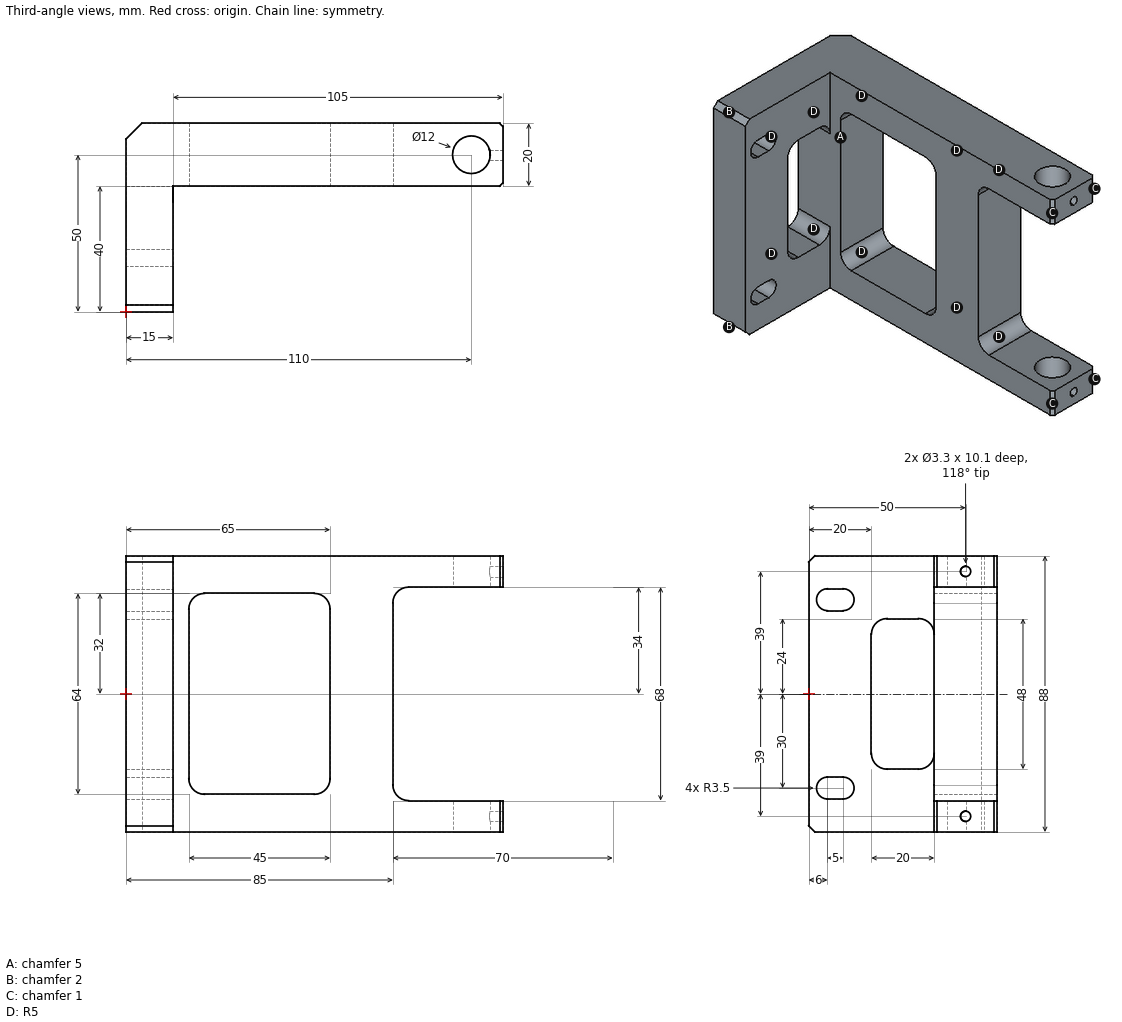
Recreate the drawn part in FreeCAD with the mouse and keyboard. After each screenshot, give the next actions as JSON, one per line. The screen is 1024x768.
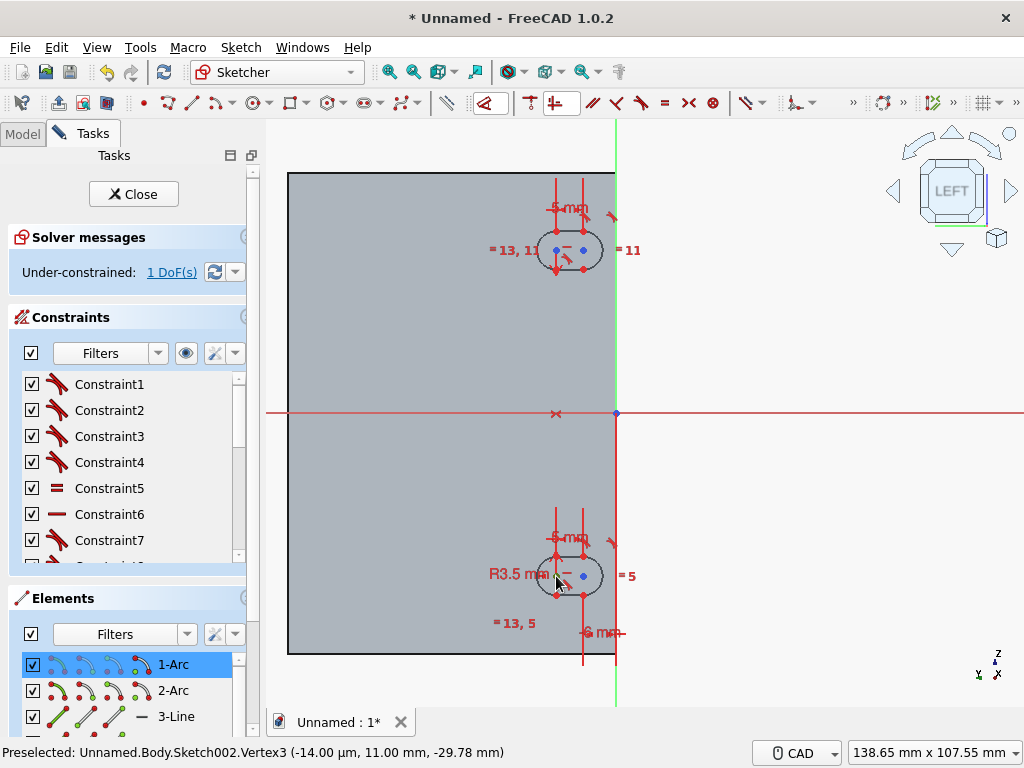
{"action": "key", "text": "i"}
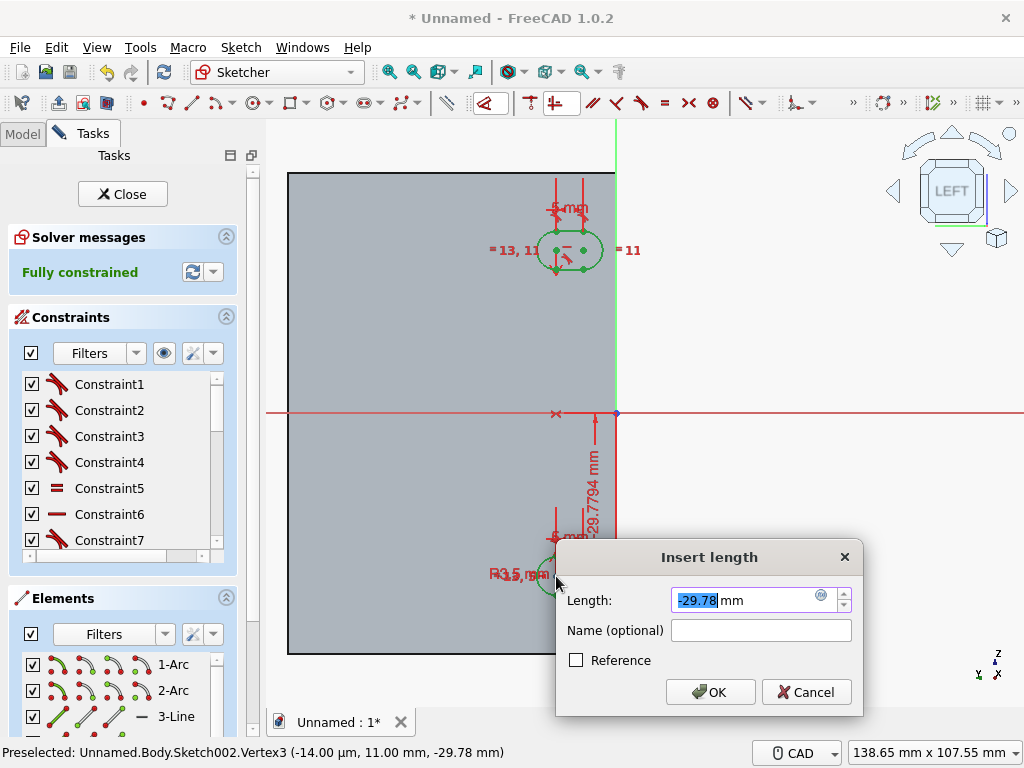
{"action": "type", "text": "-30"}
{"action": "key", "text": "Return"}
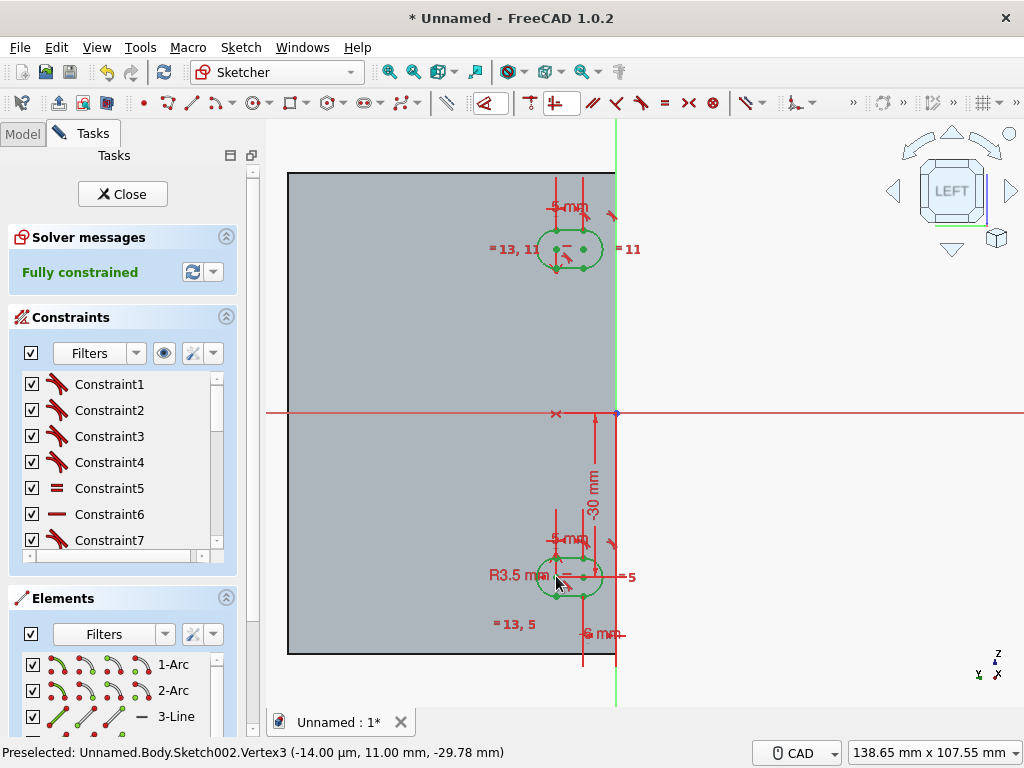
{"action": "left_click", "coordinate": [123, 194]}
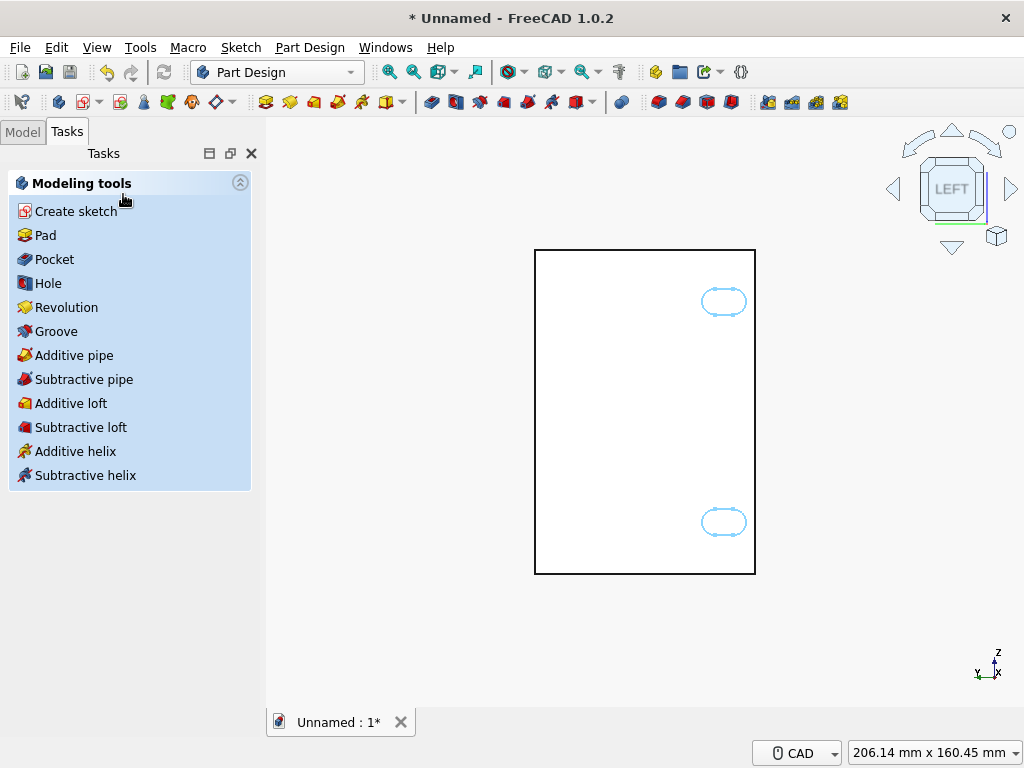
{"action": "left_click", "coordinate": [432, 102]}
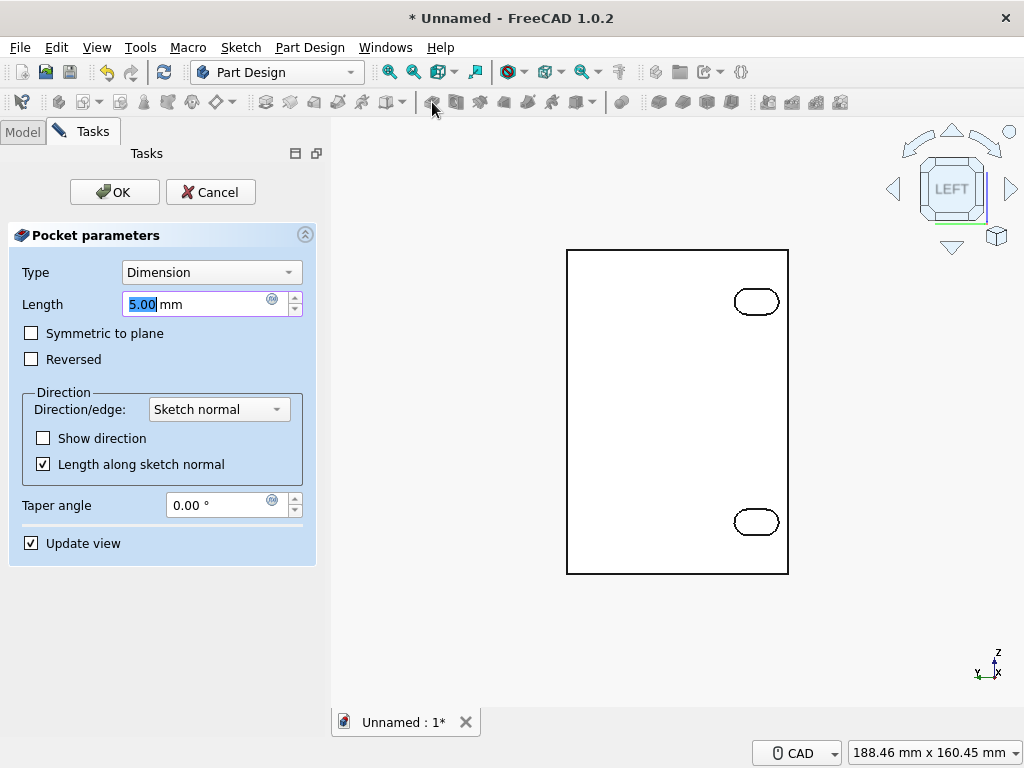
{"action": "left_click", "coordinate": [212, 272]}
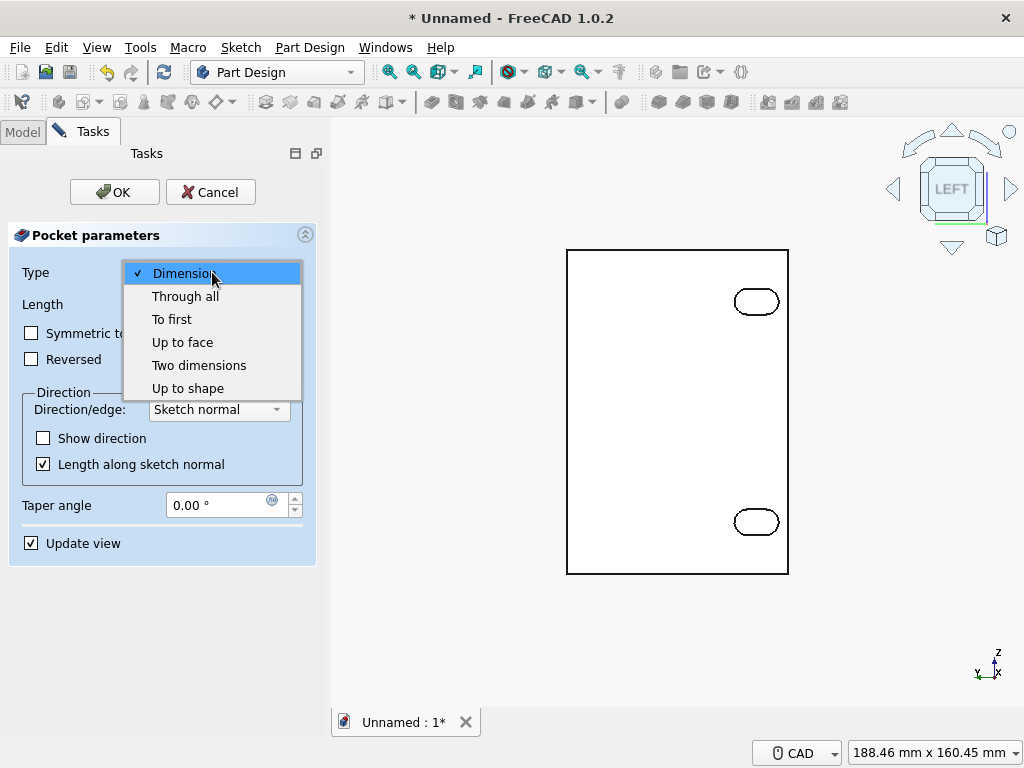
{"action": "left_click", "coordinate": [212, 296]}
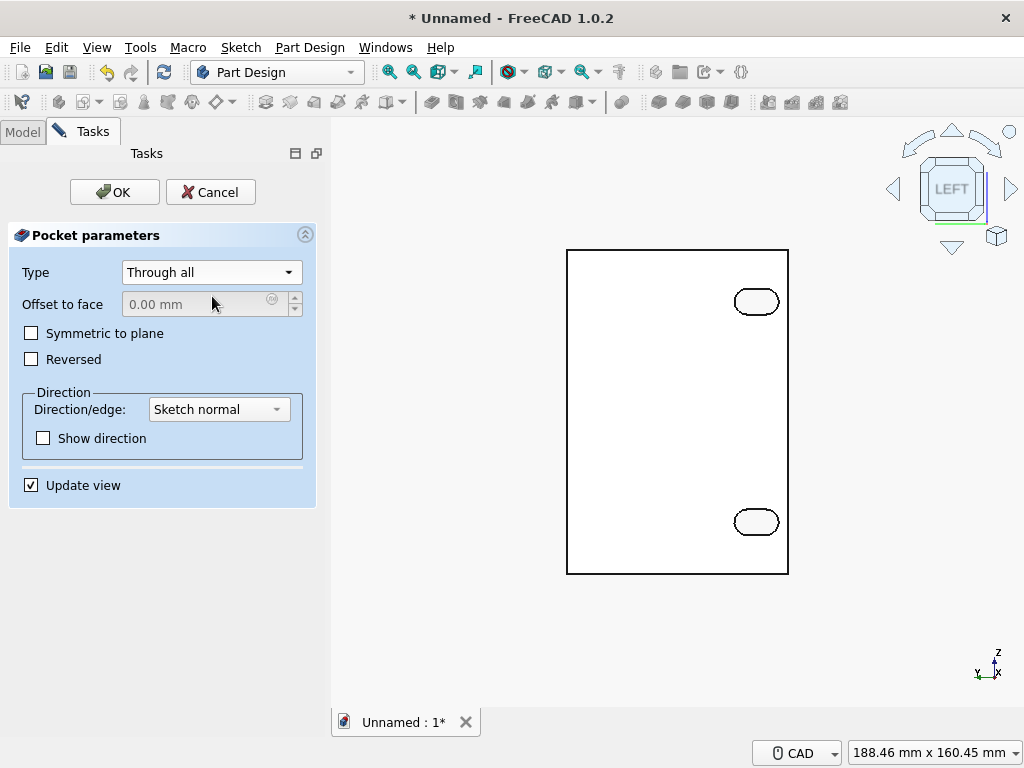
{"action": "left_click", "coordinate": [115, 192]}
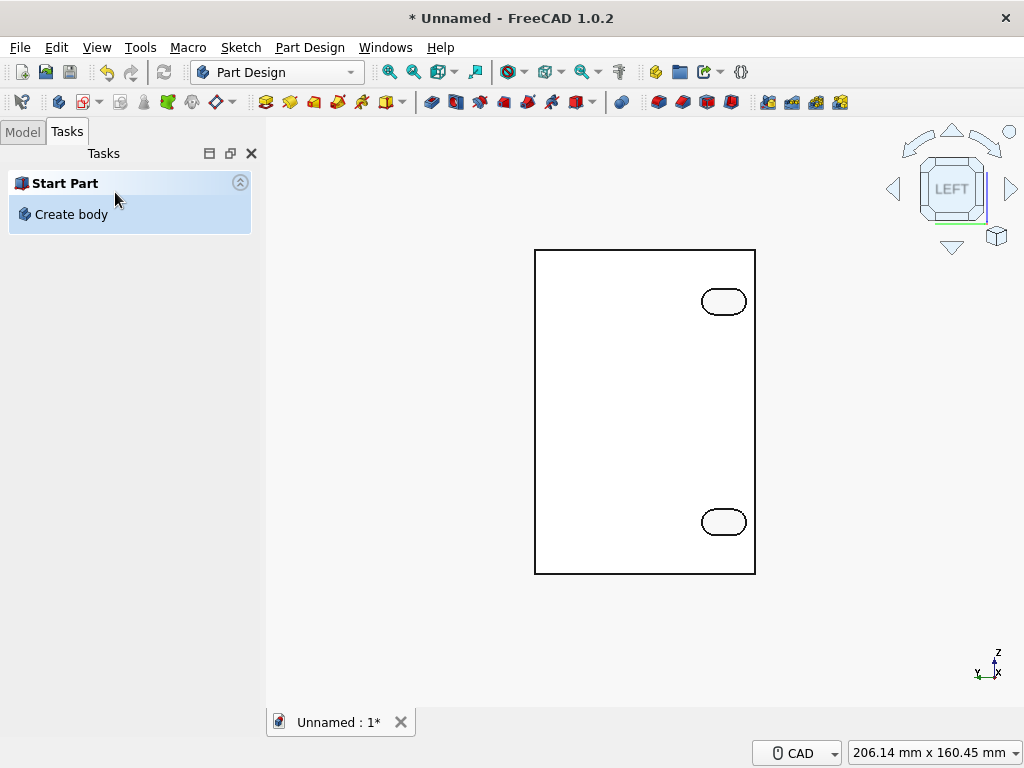
{"action": "key", "text": "0"}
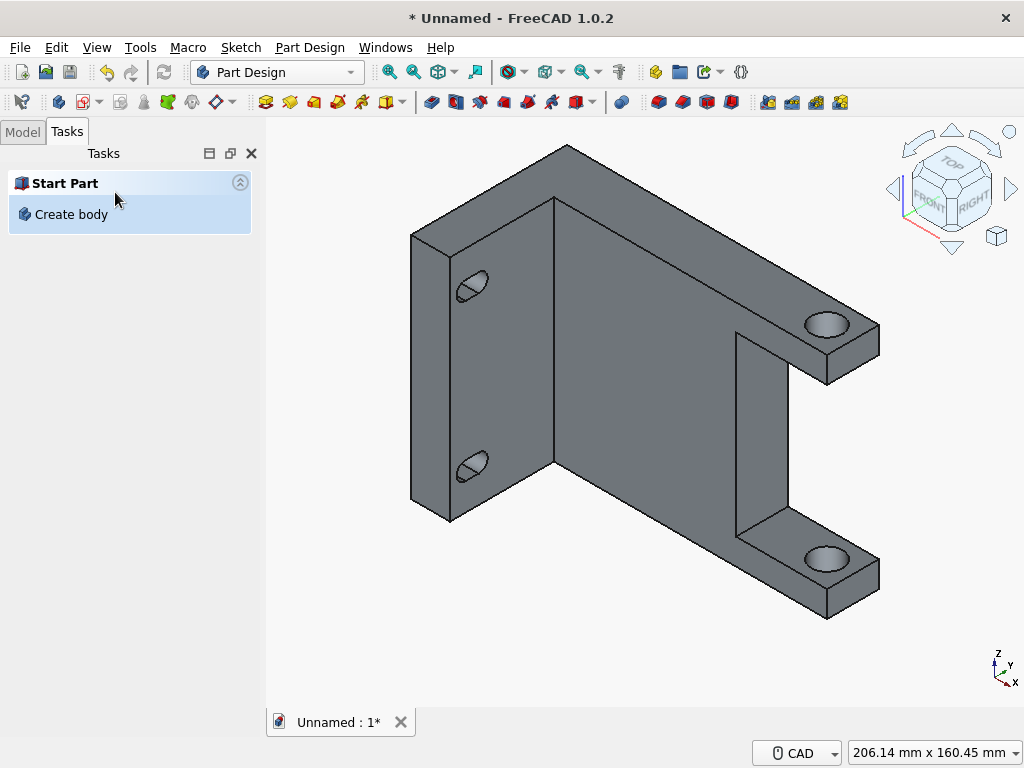
{"action": "left_click", "coordinate": [860, 584]}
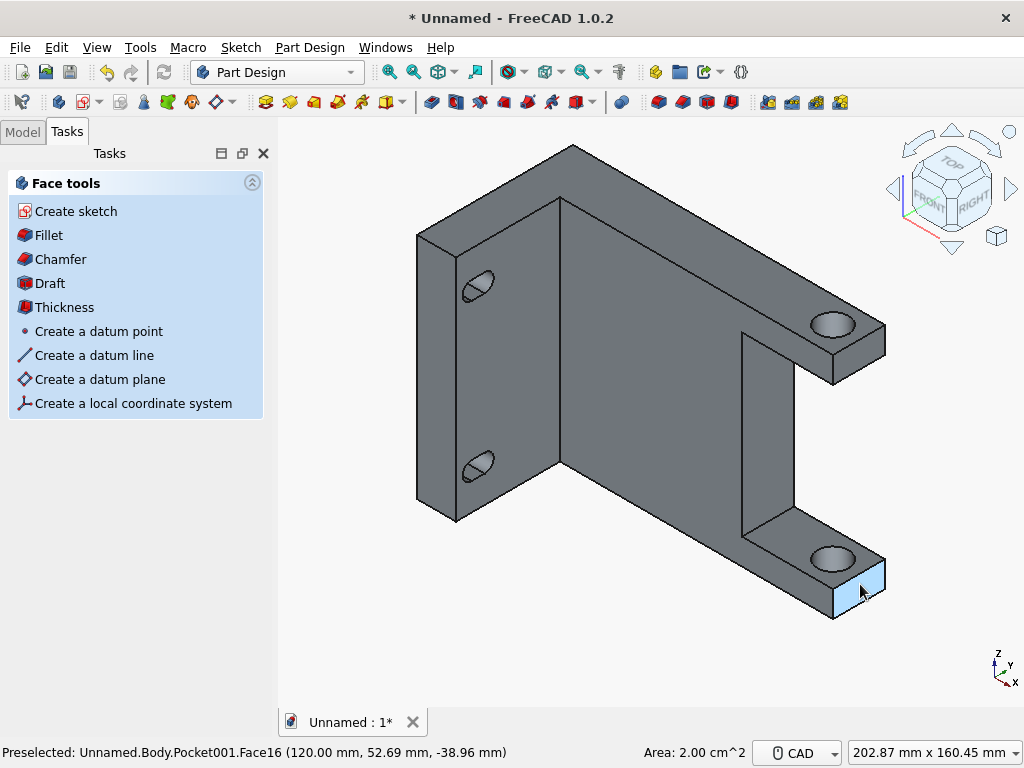
{"action": "left_click", "coordinate": [84, 102]}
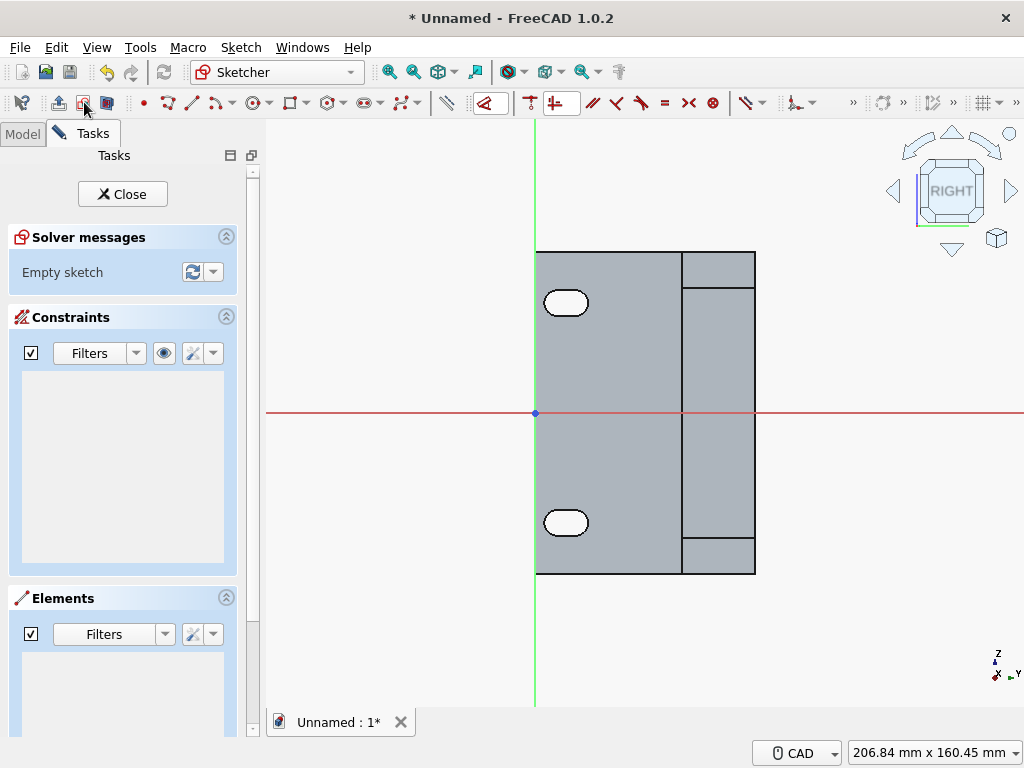
{"action": "key", "text": "g c"}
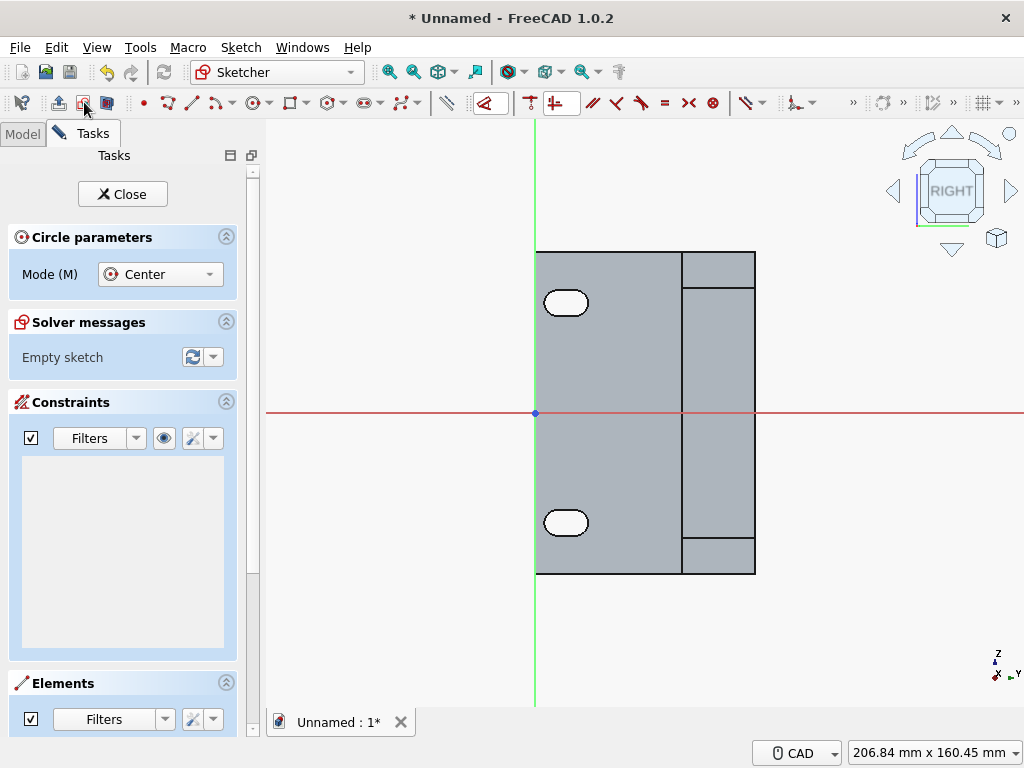
{"action": "scroll", "coordinate": [718, 270], "scroll_direction": "up", "scroll_amount": 7}